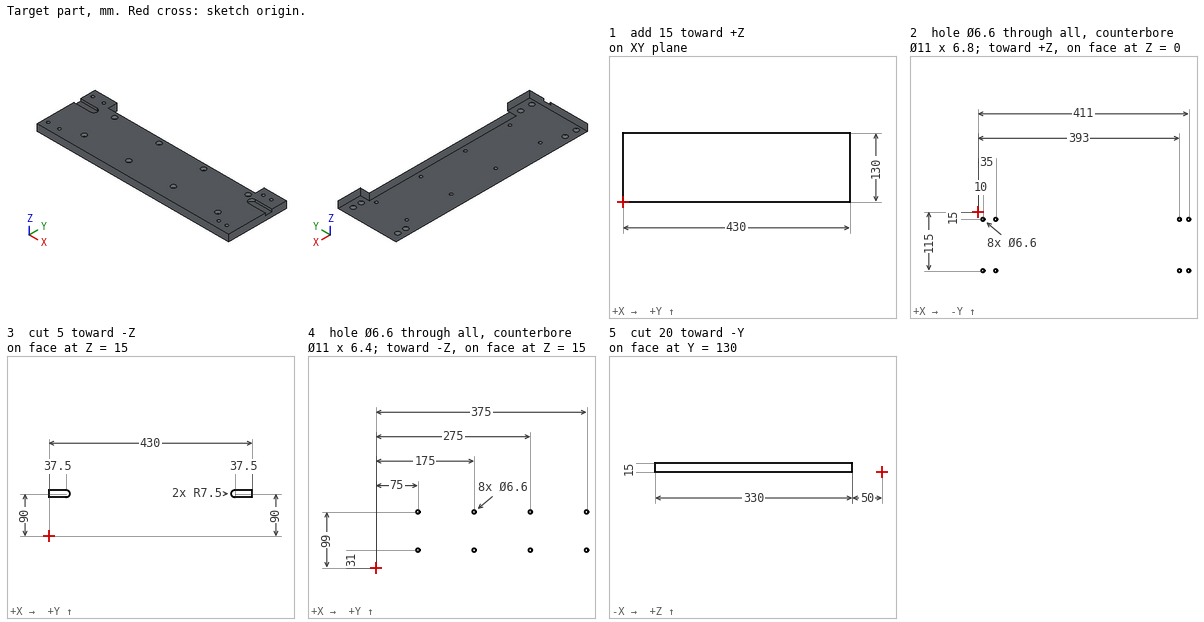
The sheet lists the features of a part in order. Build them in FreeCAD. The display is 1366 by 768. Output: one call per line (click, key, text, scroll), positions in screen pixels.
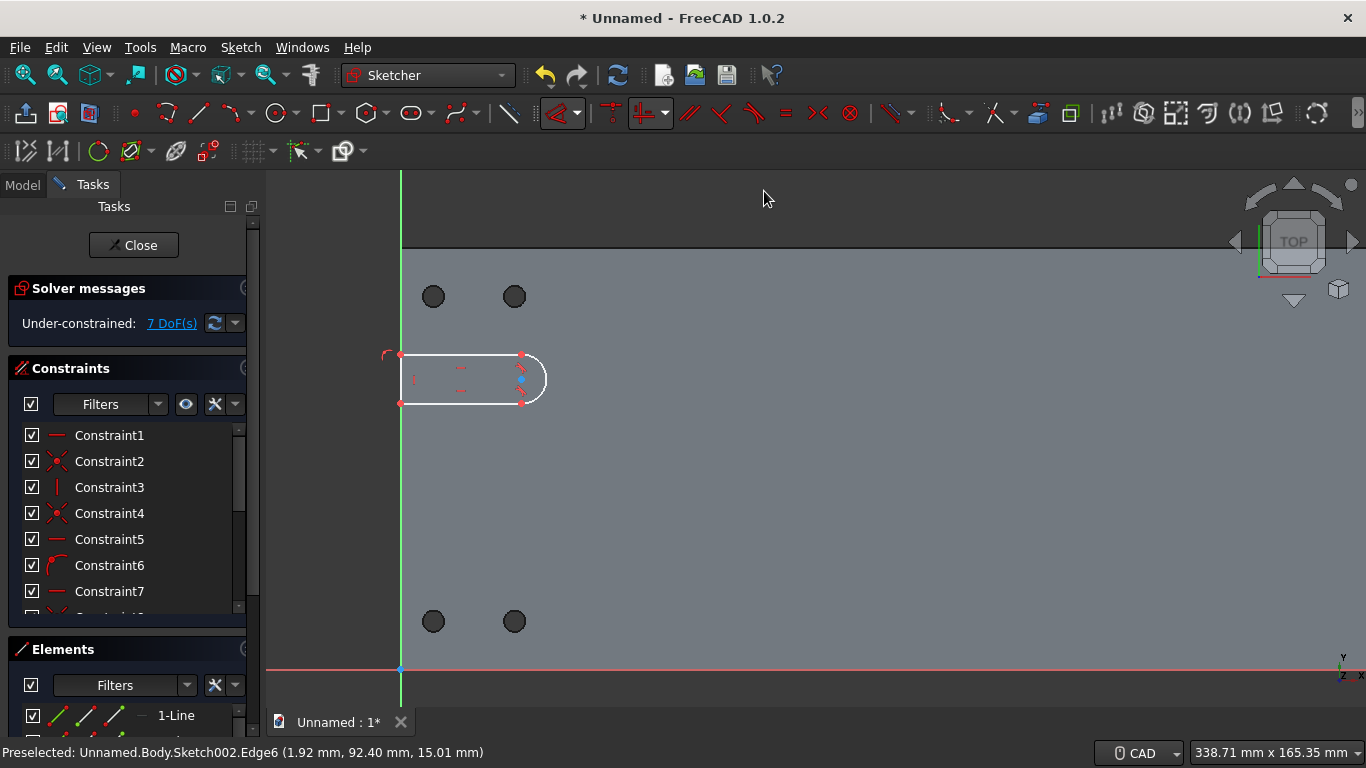
scroll(461, 379, down, 4)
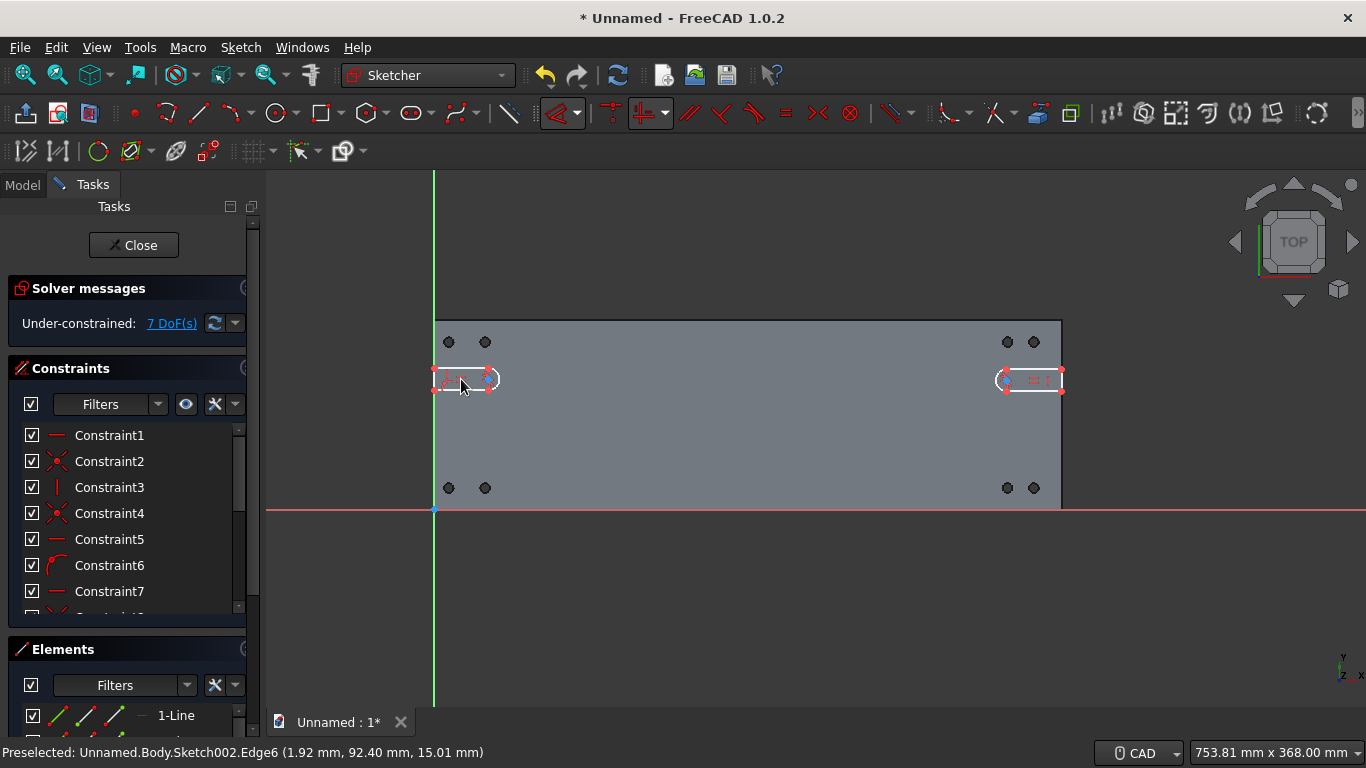
scroll(998, 374, up, 2)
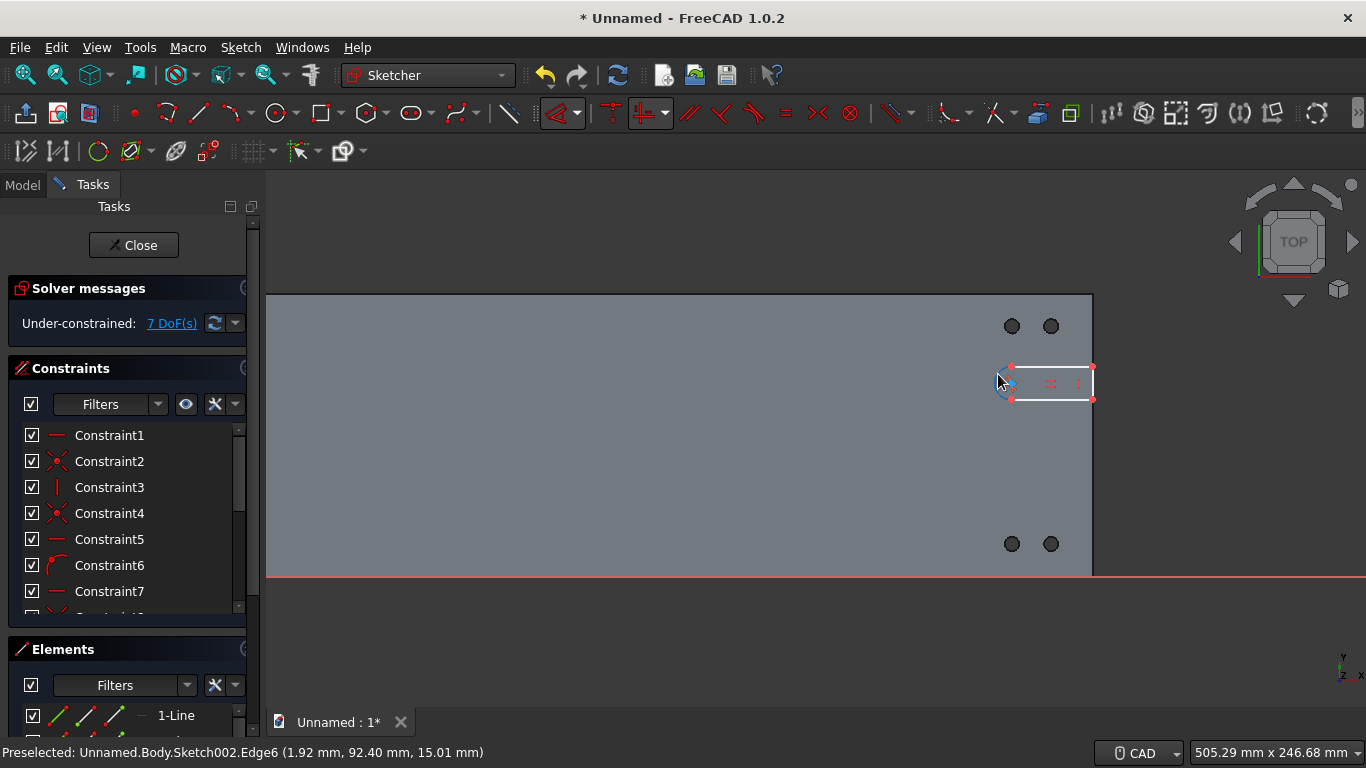
click(998, 374)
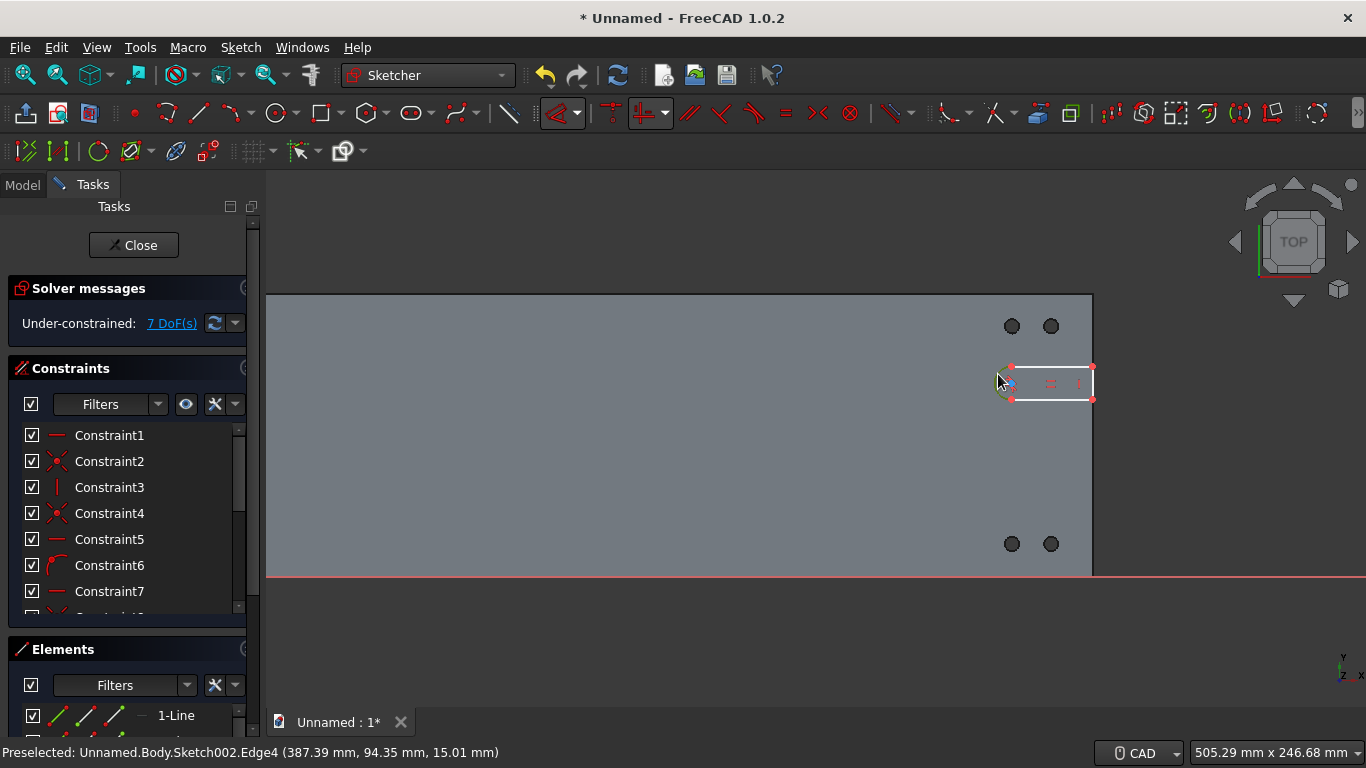
scroll(998, 373, down, 2)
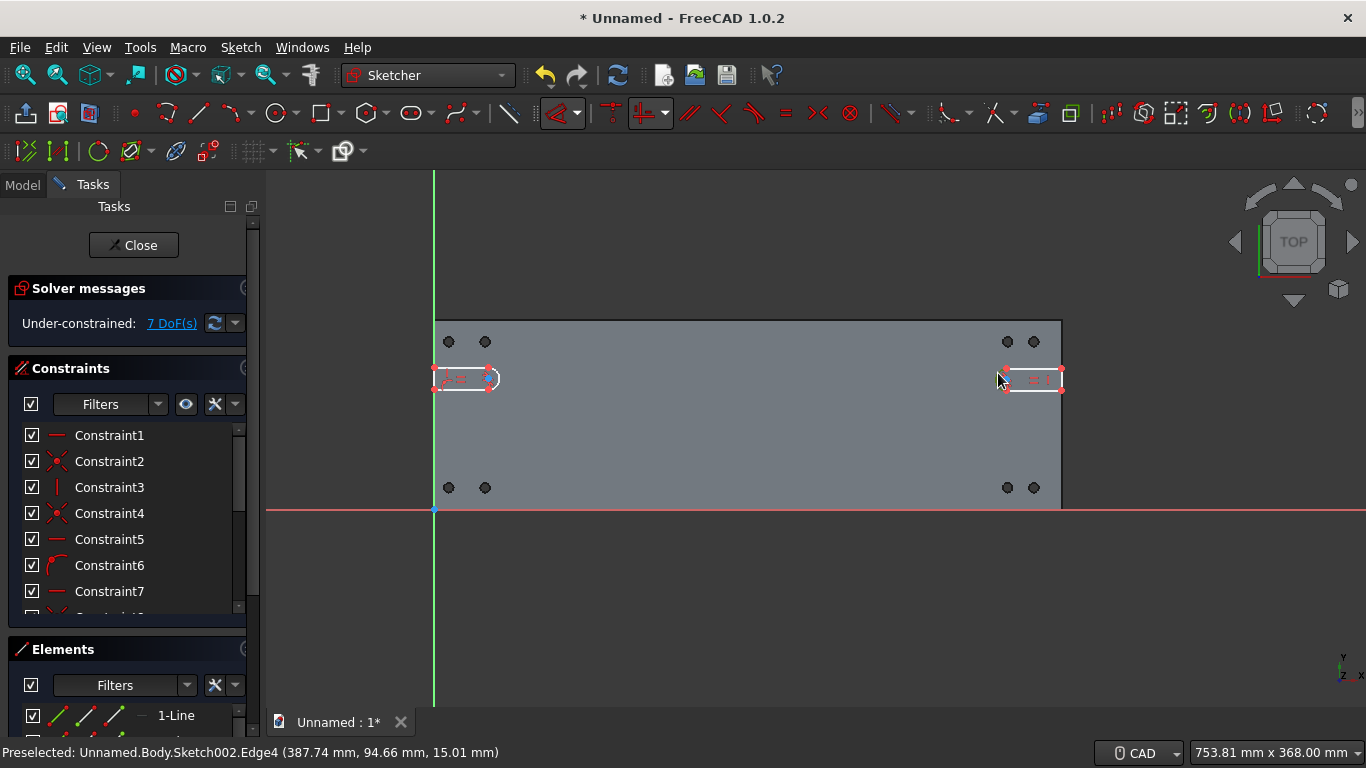
scroll(497, 385, up, 2)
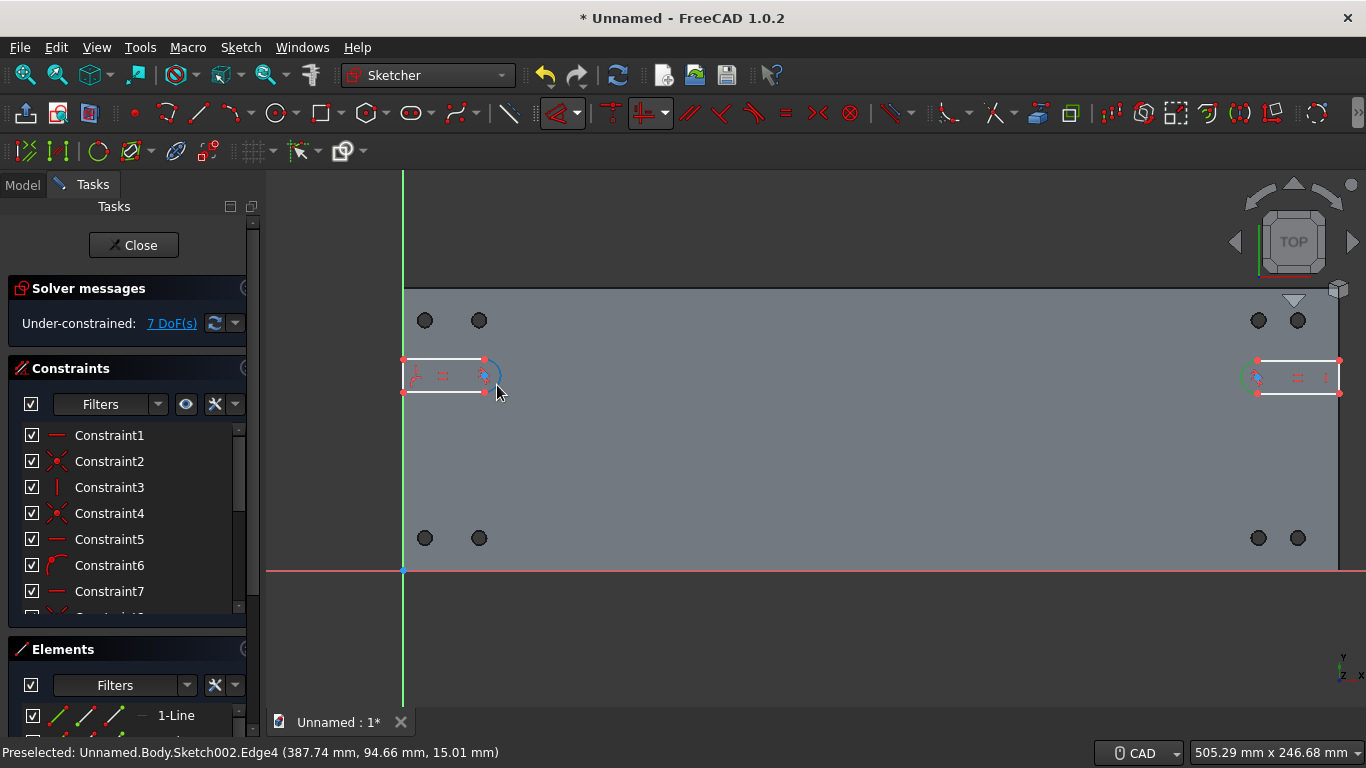
click(497, 385)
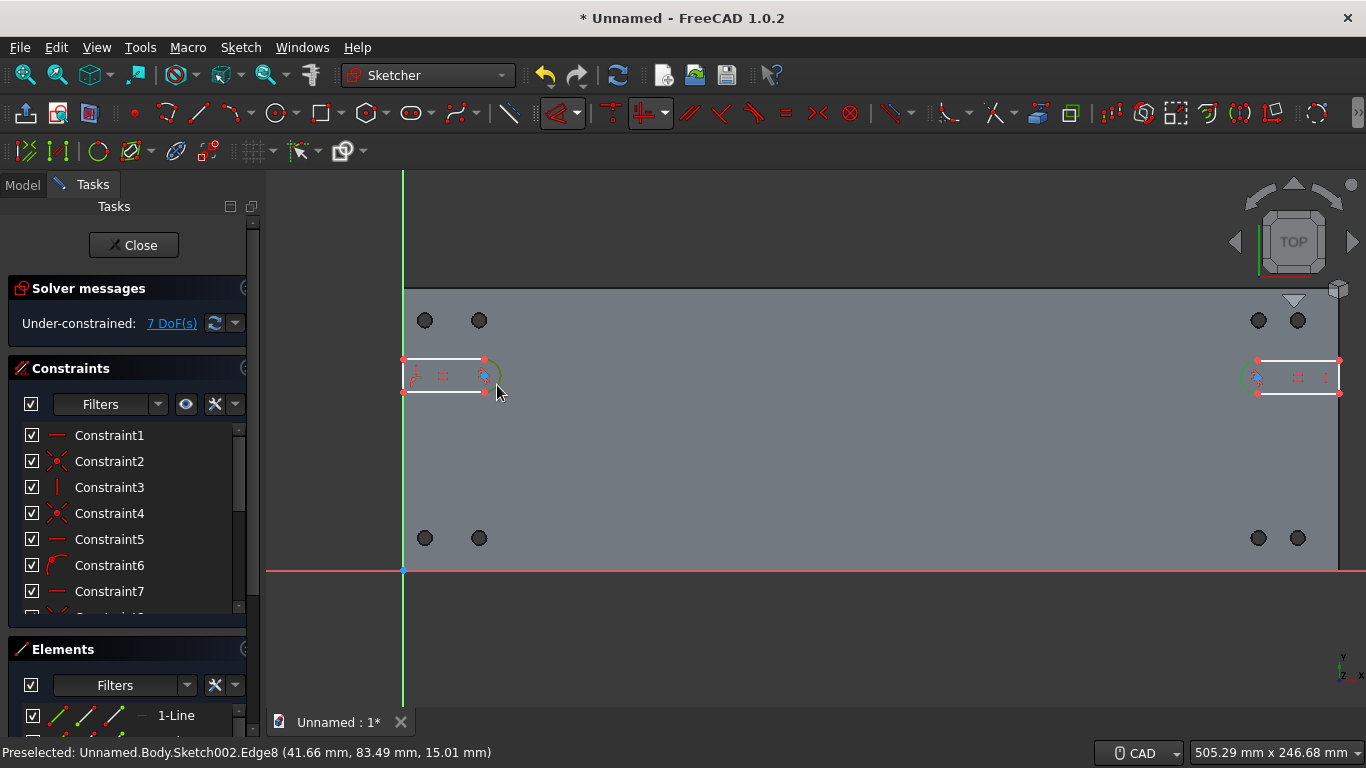
click(786, 114)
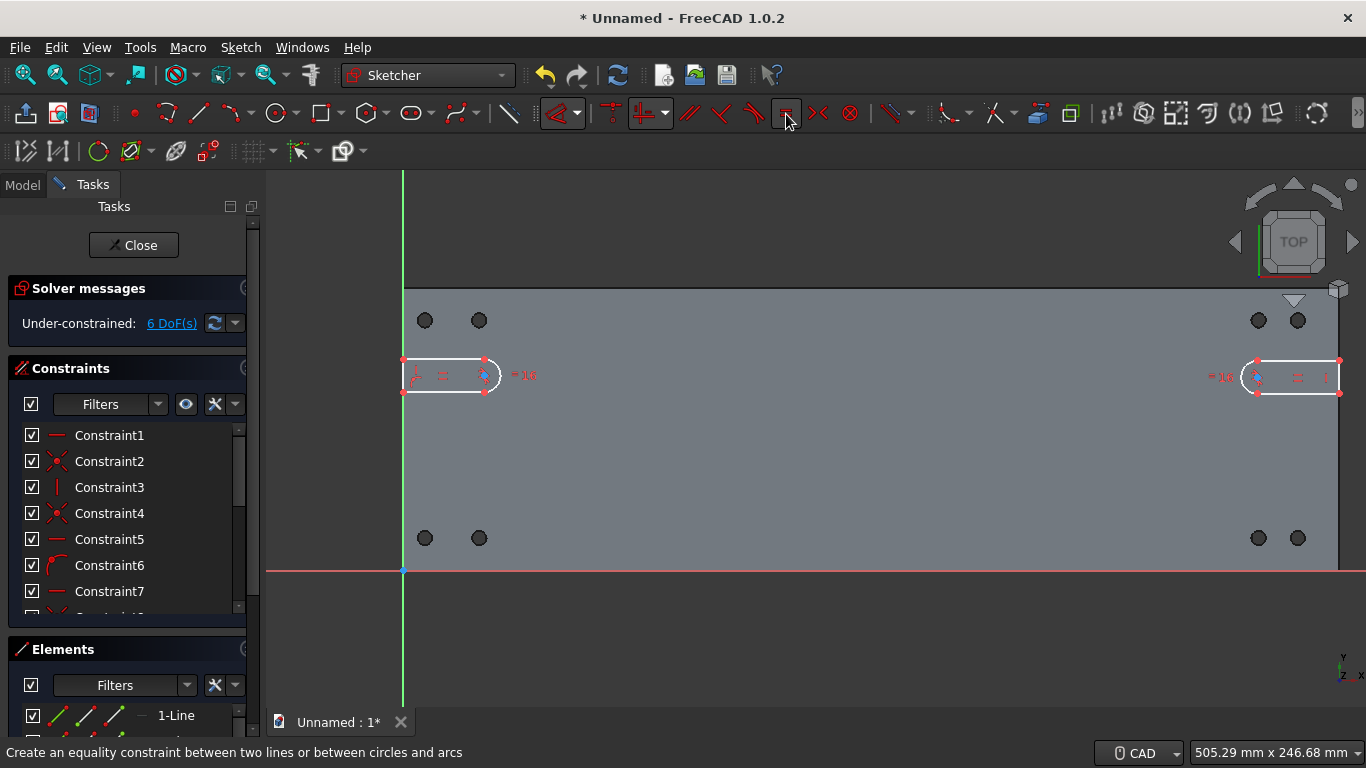
scroll(496, 385, down, 2)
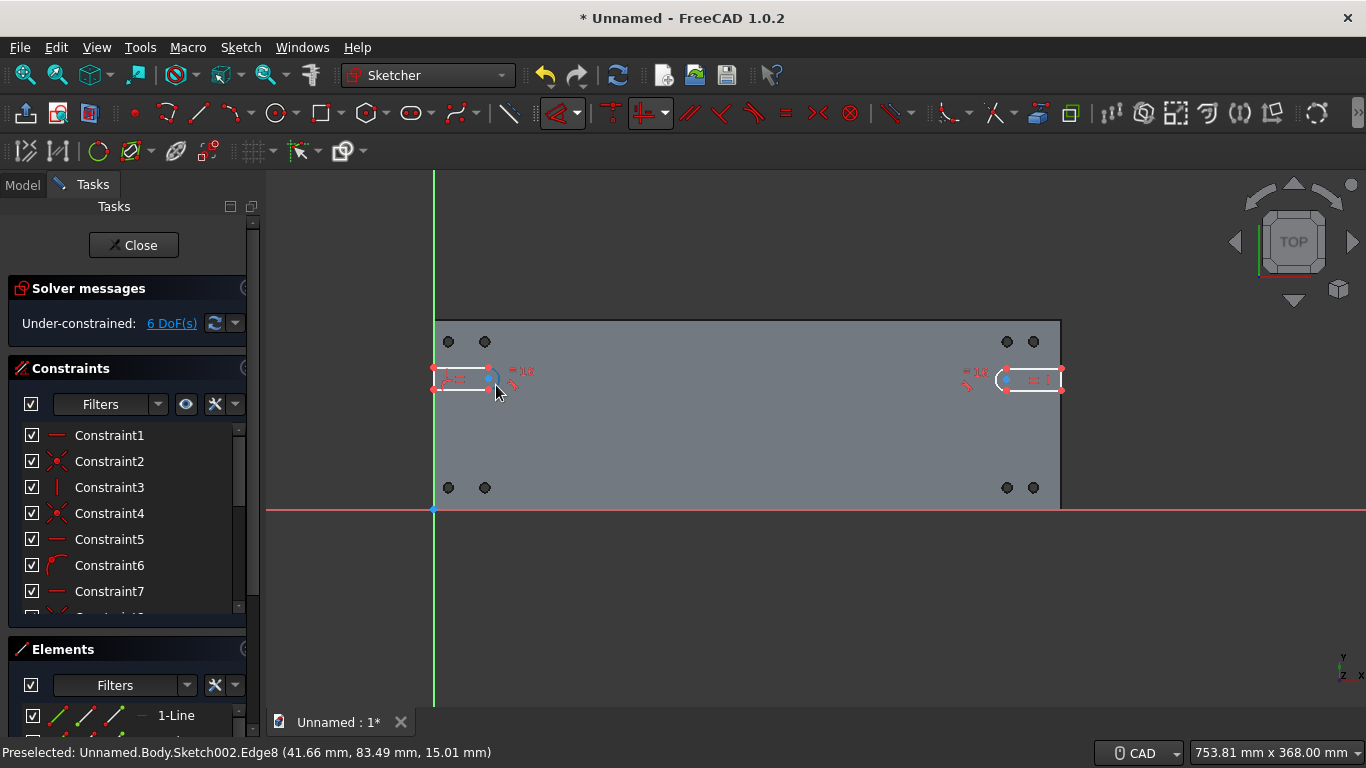
scroll(998, 374, up, 7)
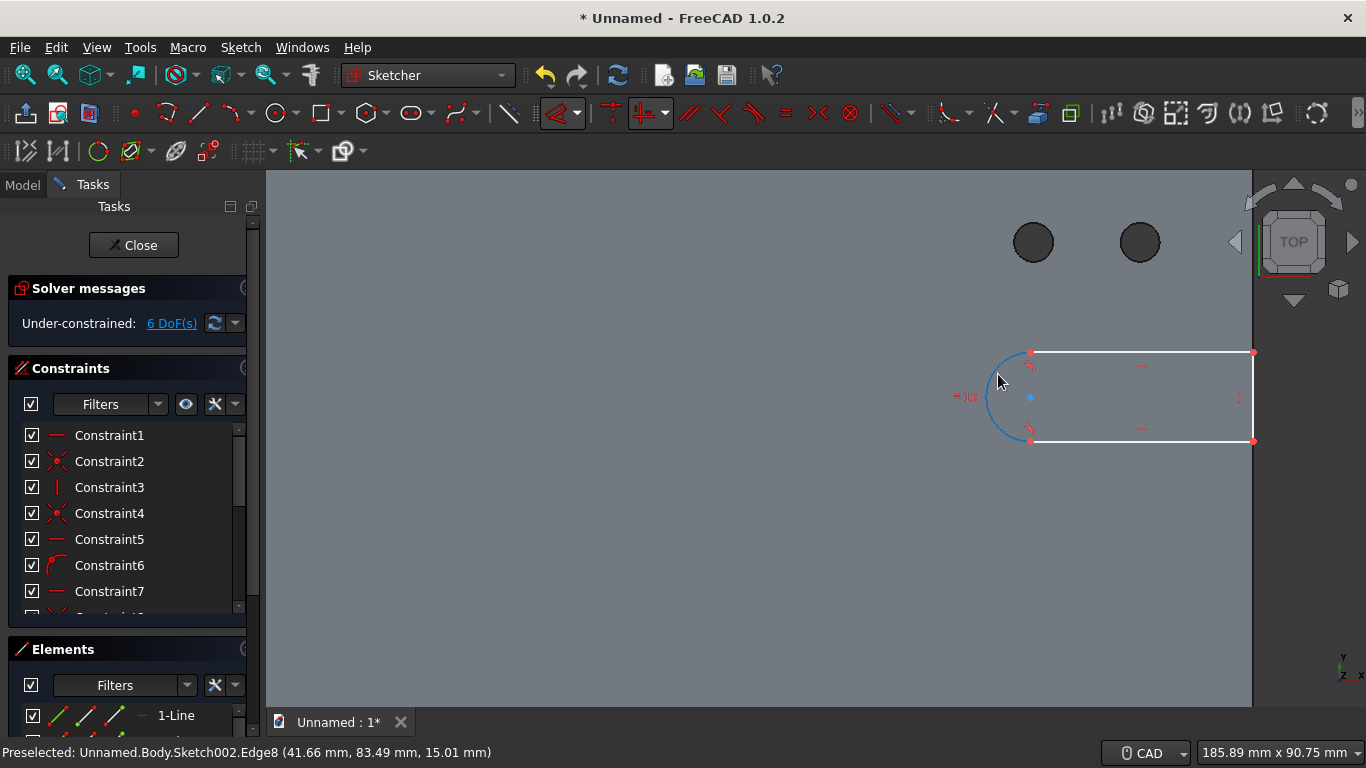
click(995, 371)